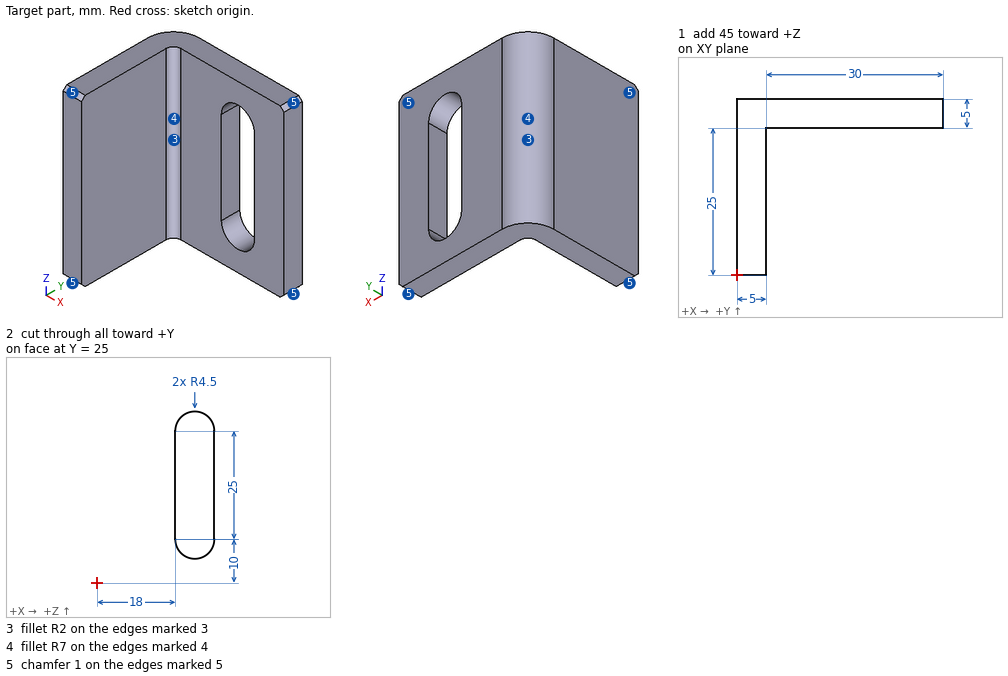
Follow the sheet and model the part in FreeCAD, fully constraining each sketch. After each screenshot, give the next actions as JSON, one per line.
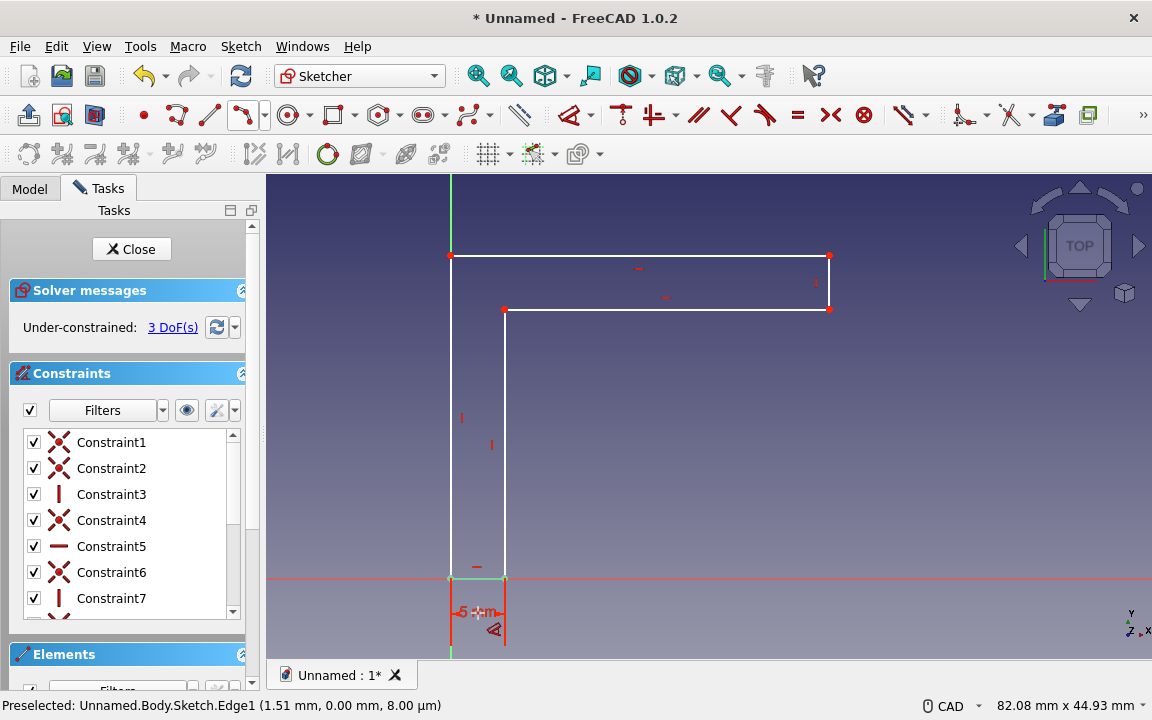
{"action": "left_click", "coordinate": [829, 294]}
{"action": "left_click", "coordinate": [863, 283]}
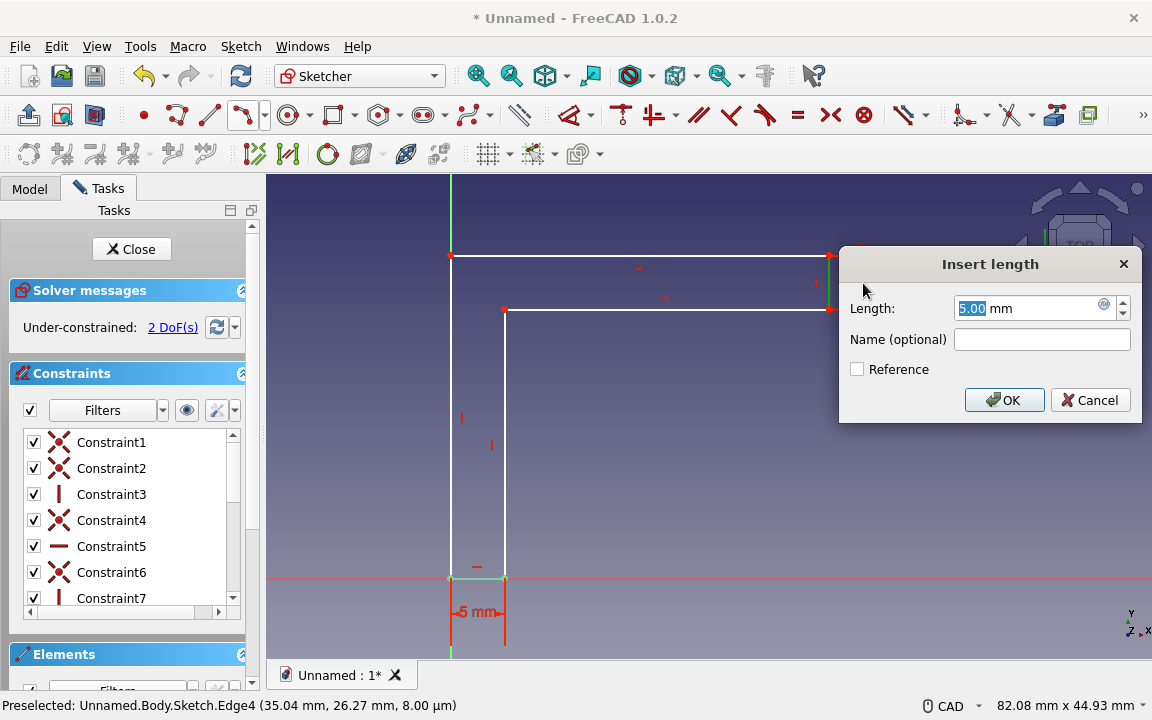
{"action": "type", "text": "5"}
{"action": "key", "text": "Return"}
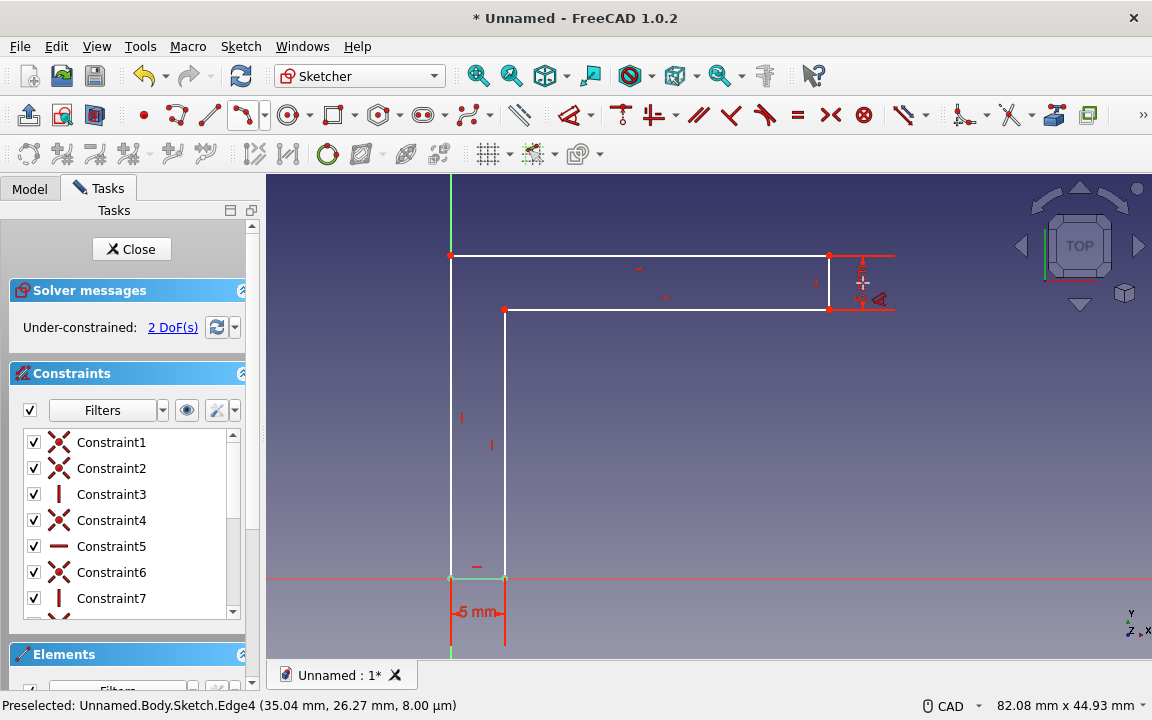
{"action": "left_click", "coordinate": [505, 498]}
{"action": "left_click", "coordinate": [471, 444]}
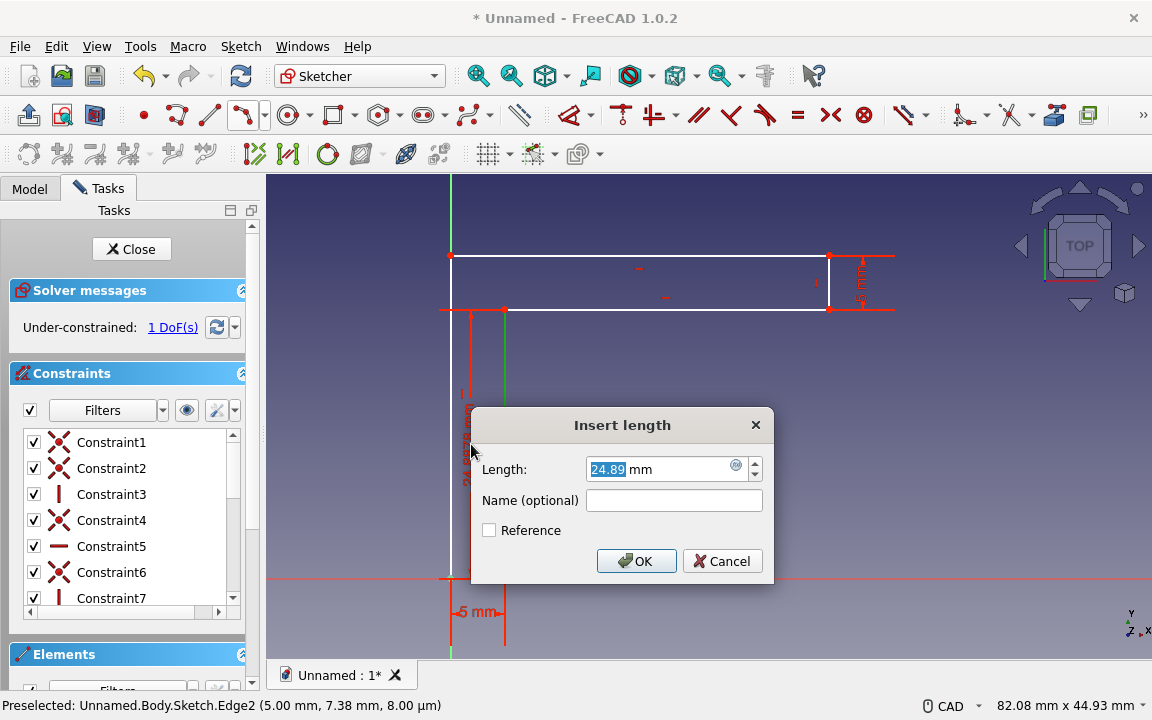
{"action": "type", "text": "25"}
{"action": "key", "text": "Return"}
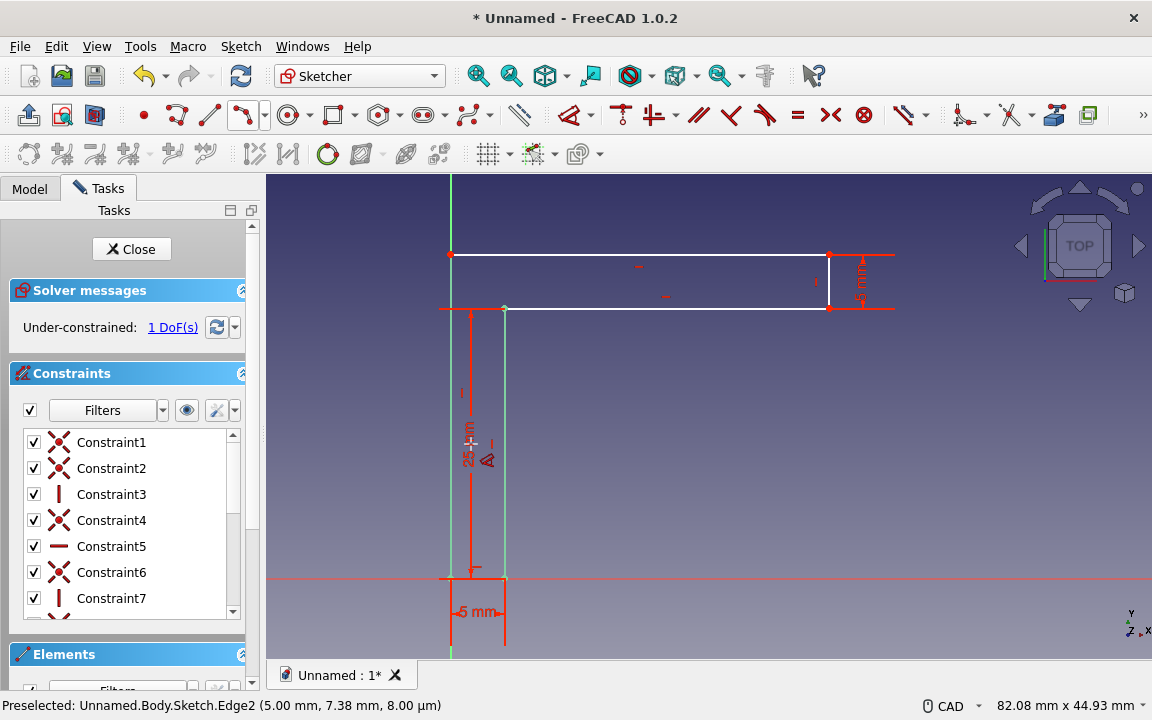
{"action": "left_click", "coordinate": [602, 309]}
{"action": "left_click", "coordinate": [667, 275]}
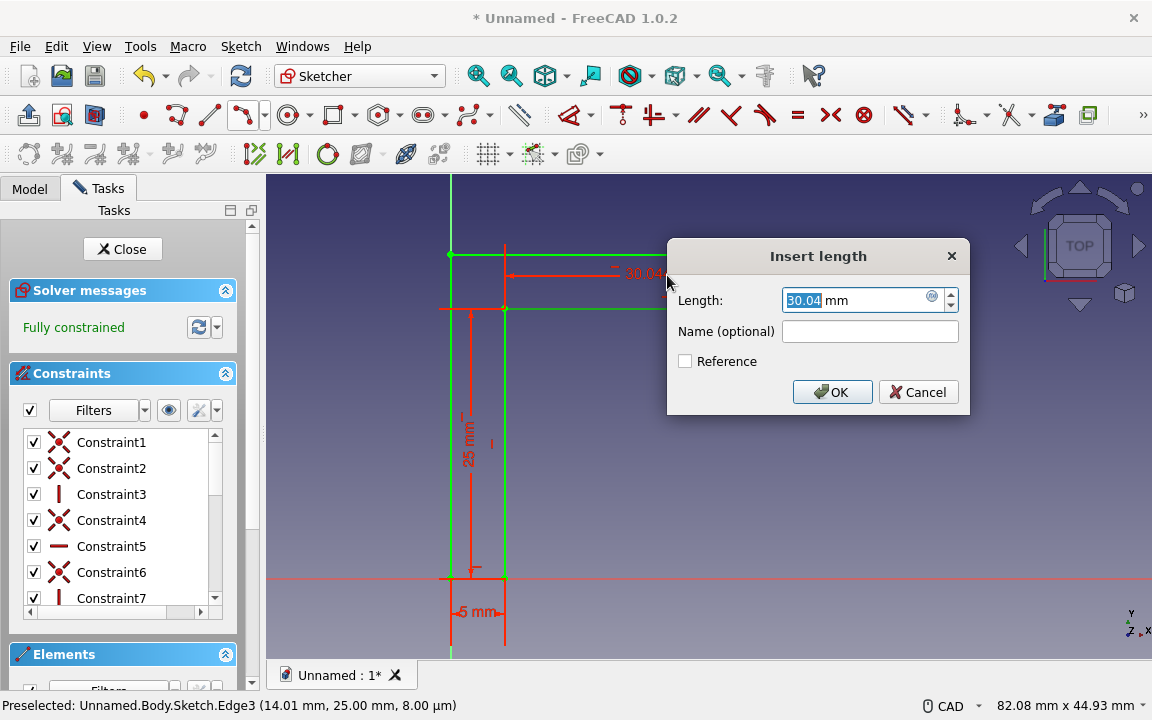
{"action": "type", "text": "30"}
{"action": "key", "text": "Return"}
{"action": "key", "text": "Escape"}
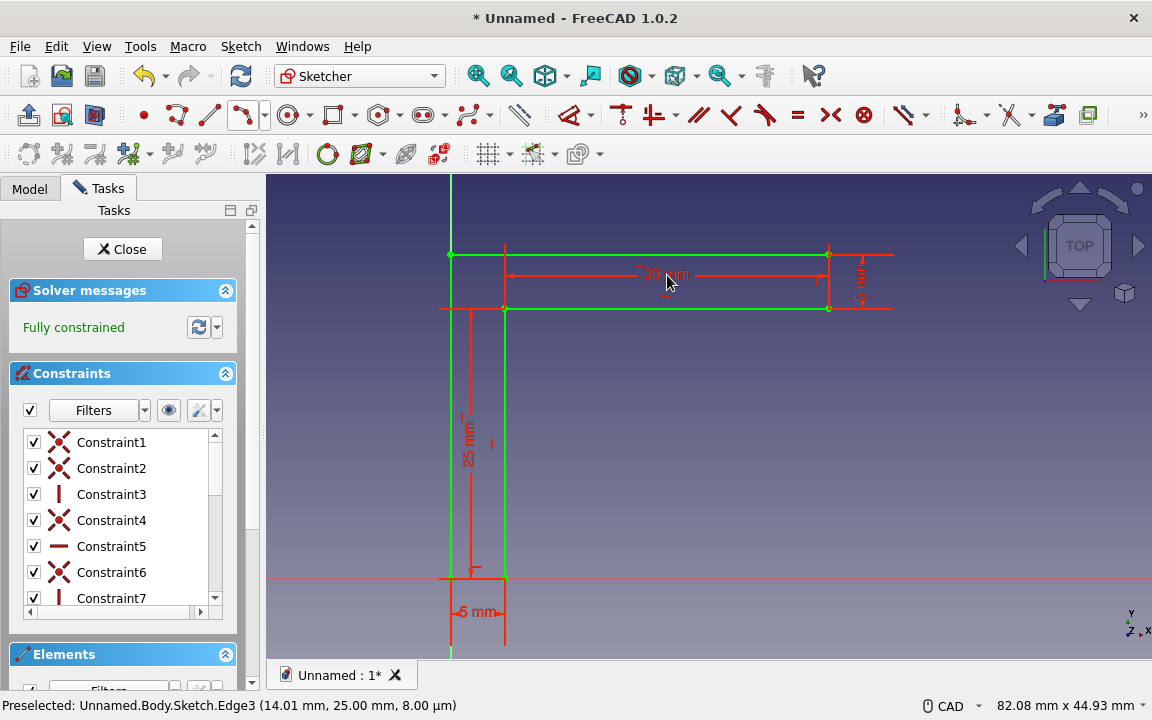
{"action": "left_click", "coordinate": [123, 249]}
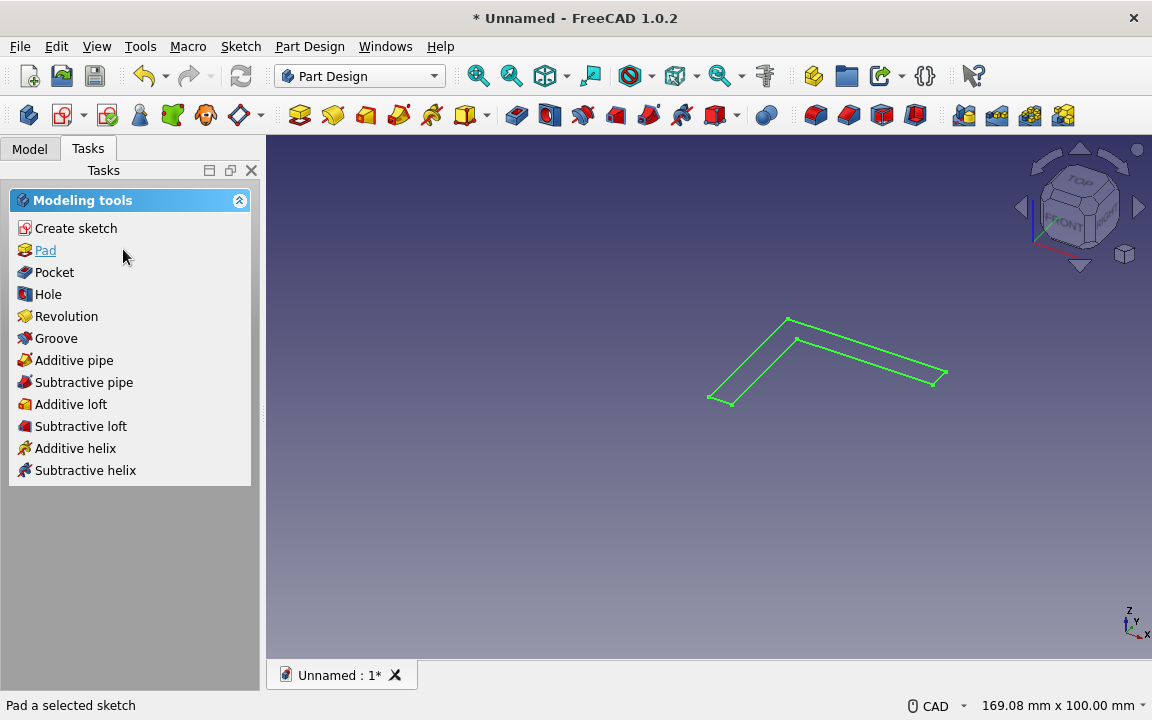
{"action": "left_click", "coordinate": [300, 116]}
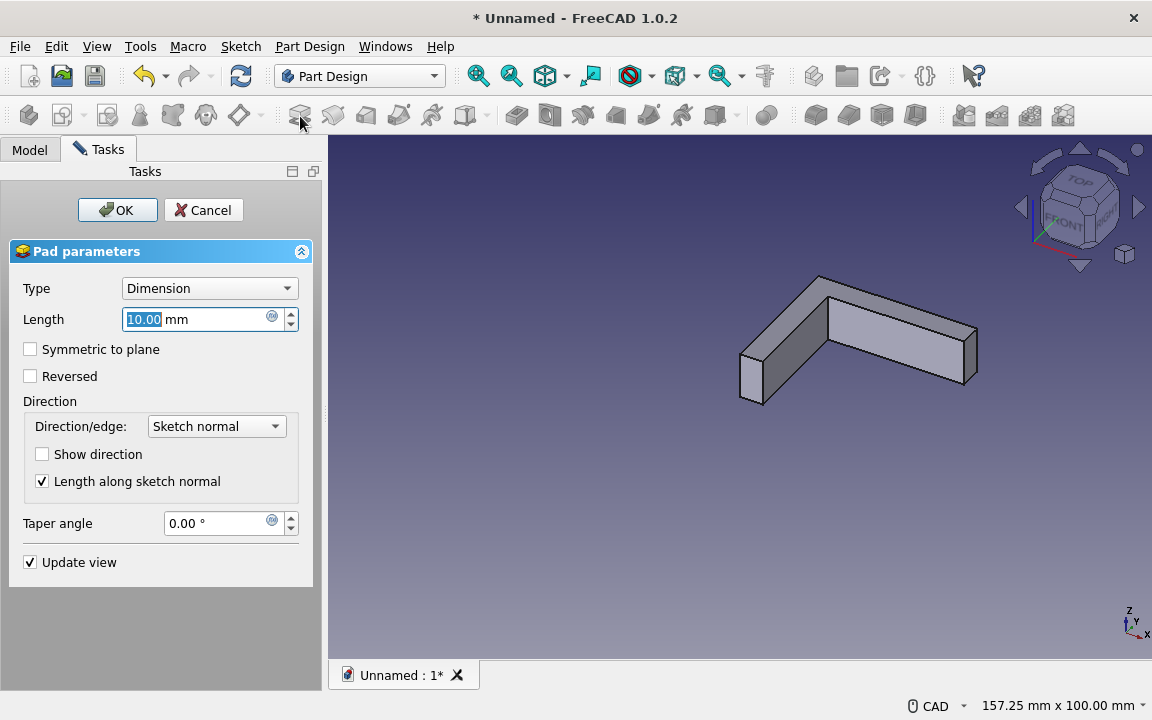
{"action": "type", "text": "45"}
{"action": "key", "text": "Tab"}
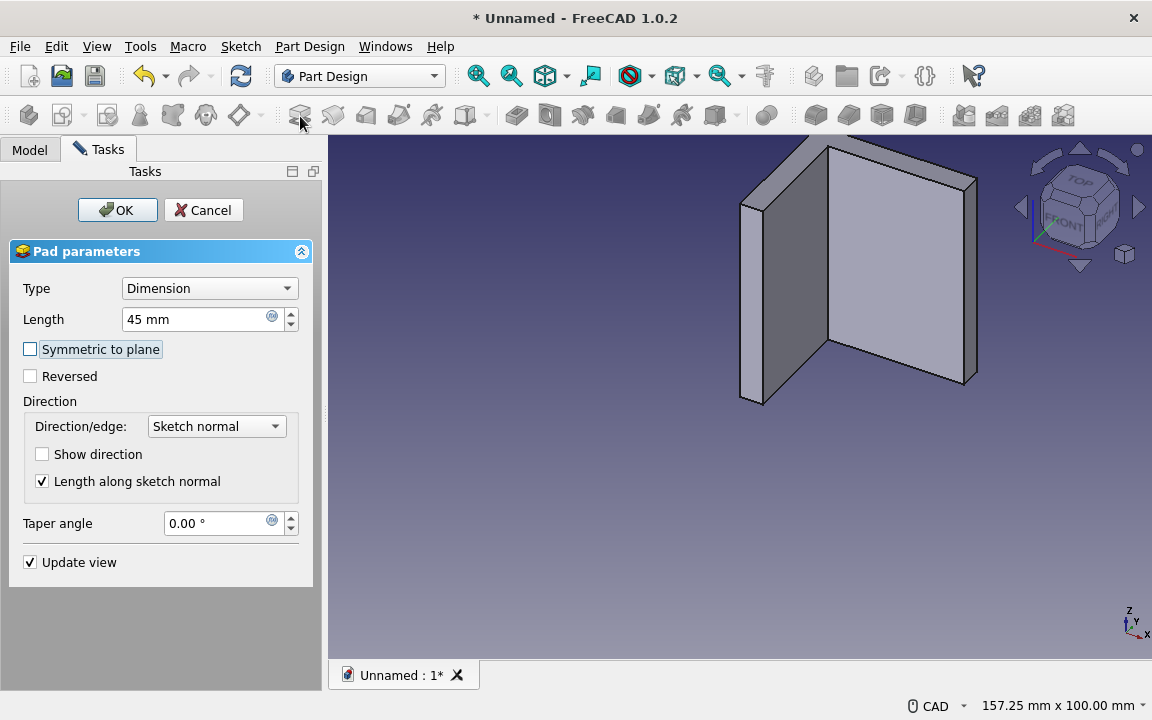
{"action": "left_click", "coordinate": [118, 210]}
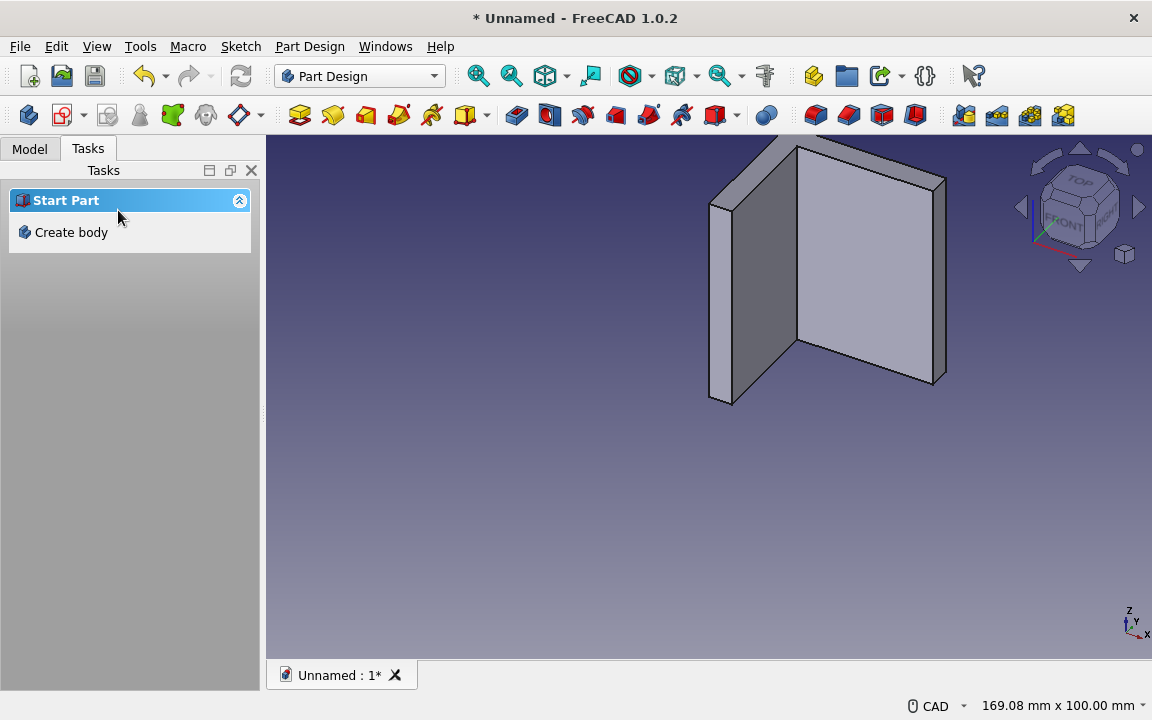
{"action": "key", "text": "v f"}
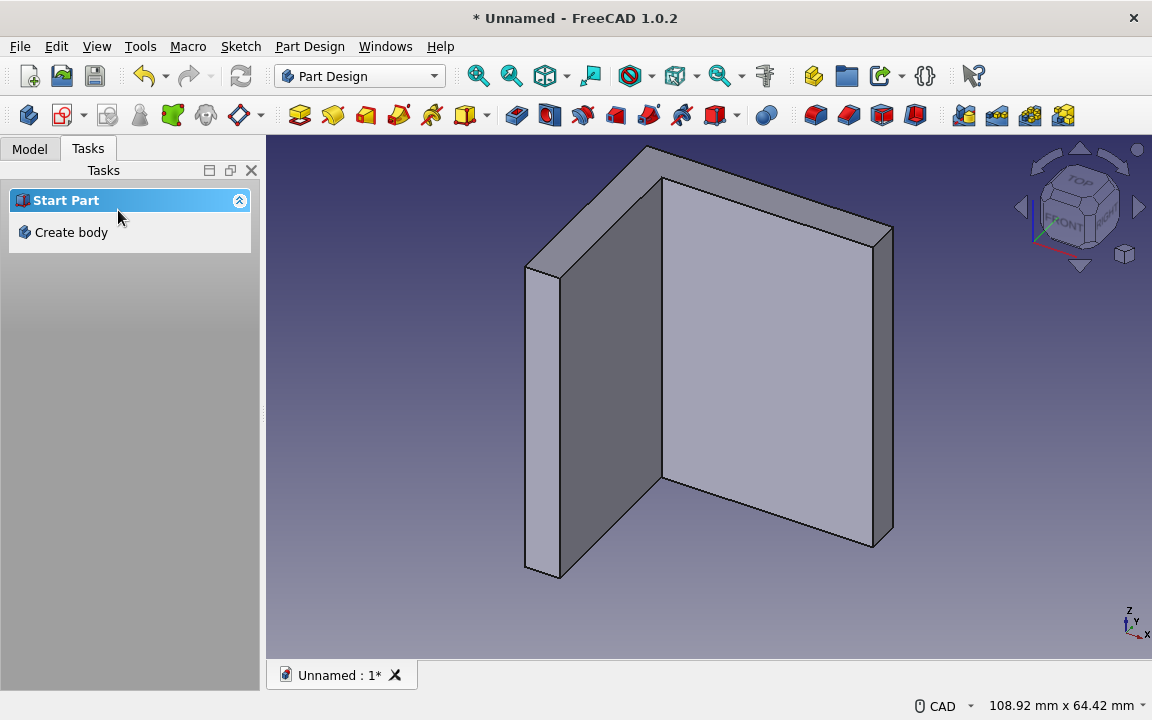
{"action": "left_click", "coordinate": [767, 319]}